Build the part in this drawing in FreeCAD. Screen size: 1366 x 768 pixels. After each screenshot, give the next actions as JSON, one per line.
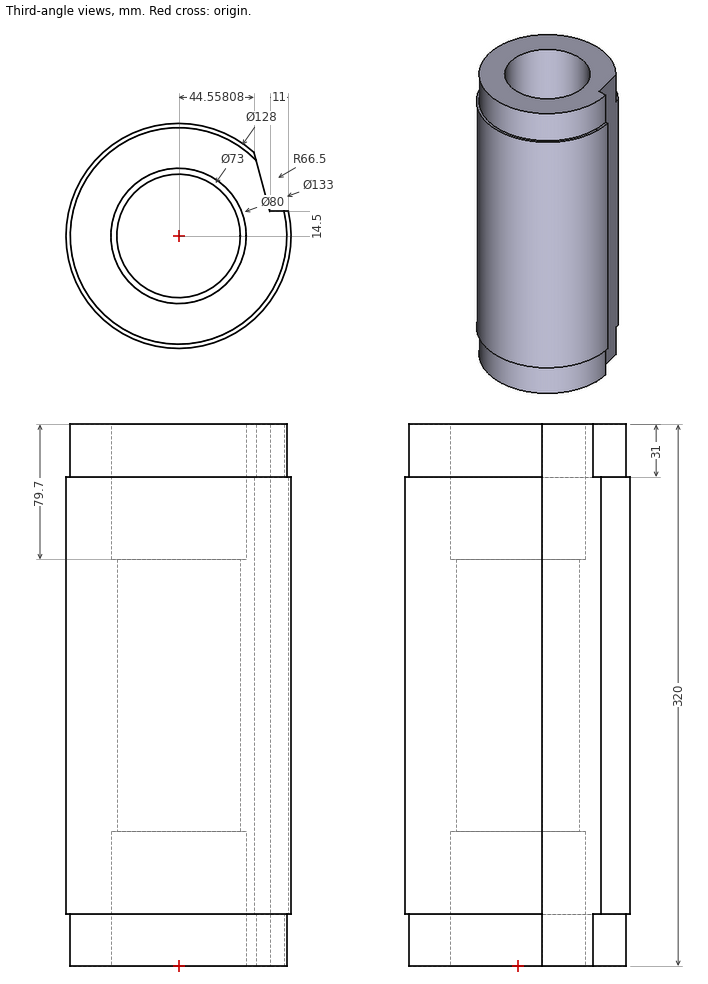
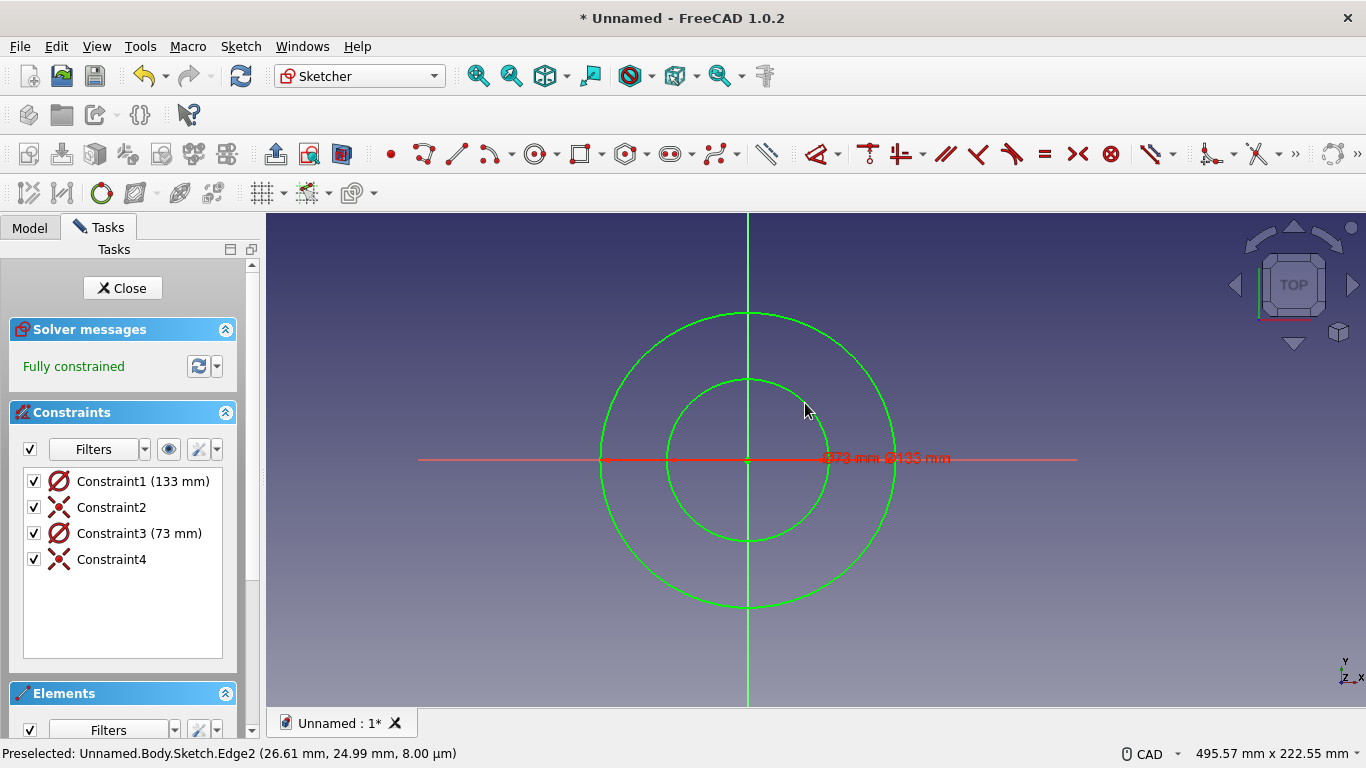
{"action": "left_click", "coordinate": [123, 288]}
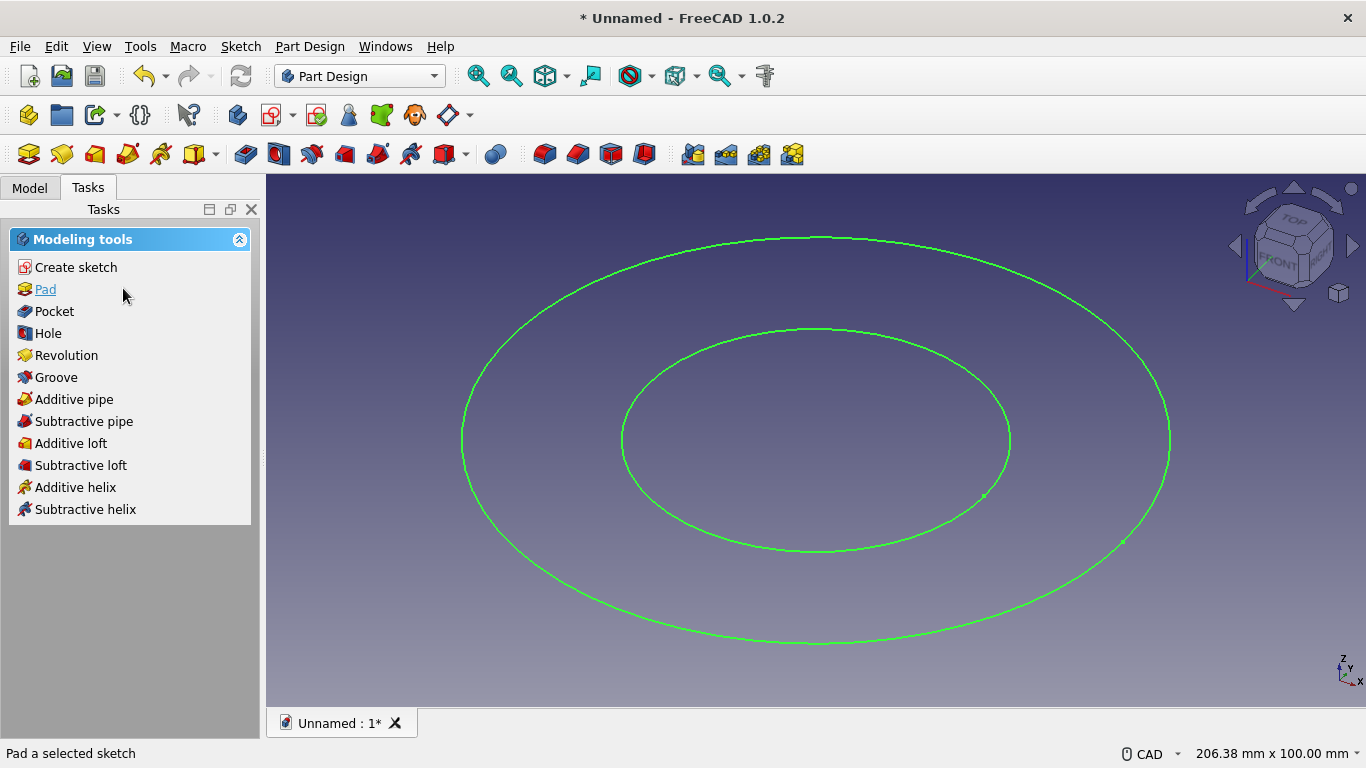
{"action": "left_click", "coordinate": [29, 154]}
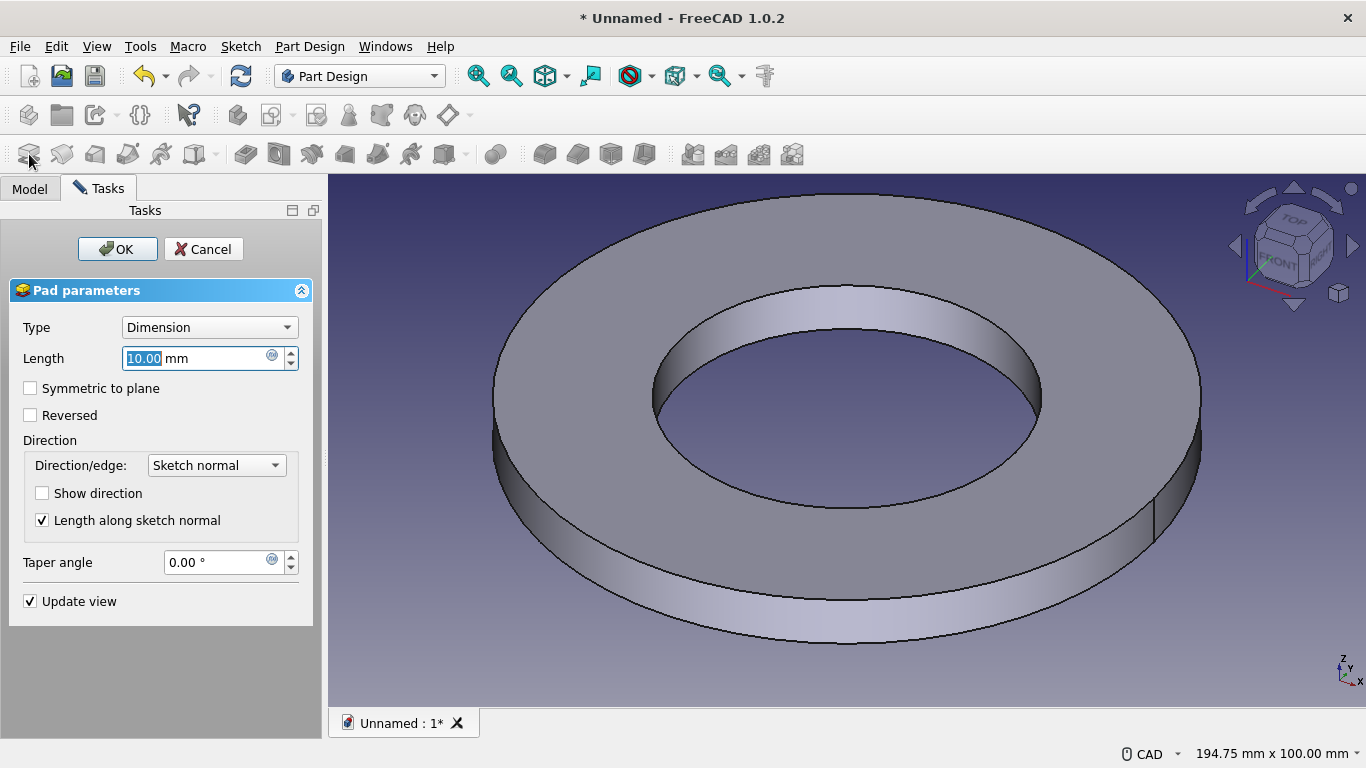
{"action": "type", "text": "320"}
{"action": "key", "text": "Tab"}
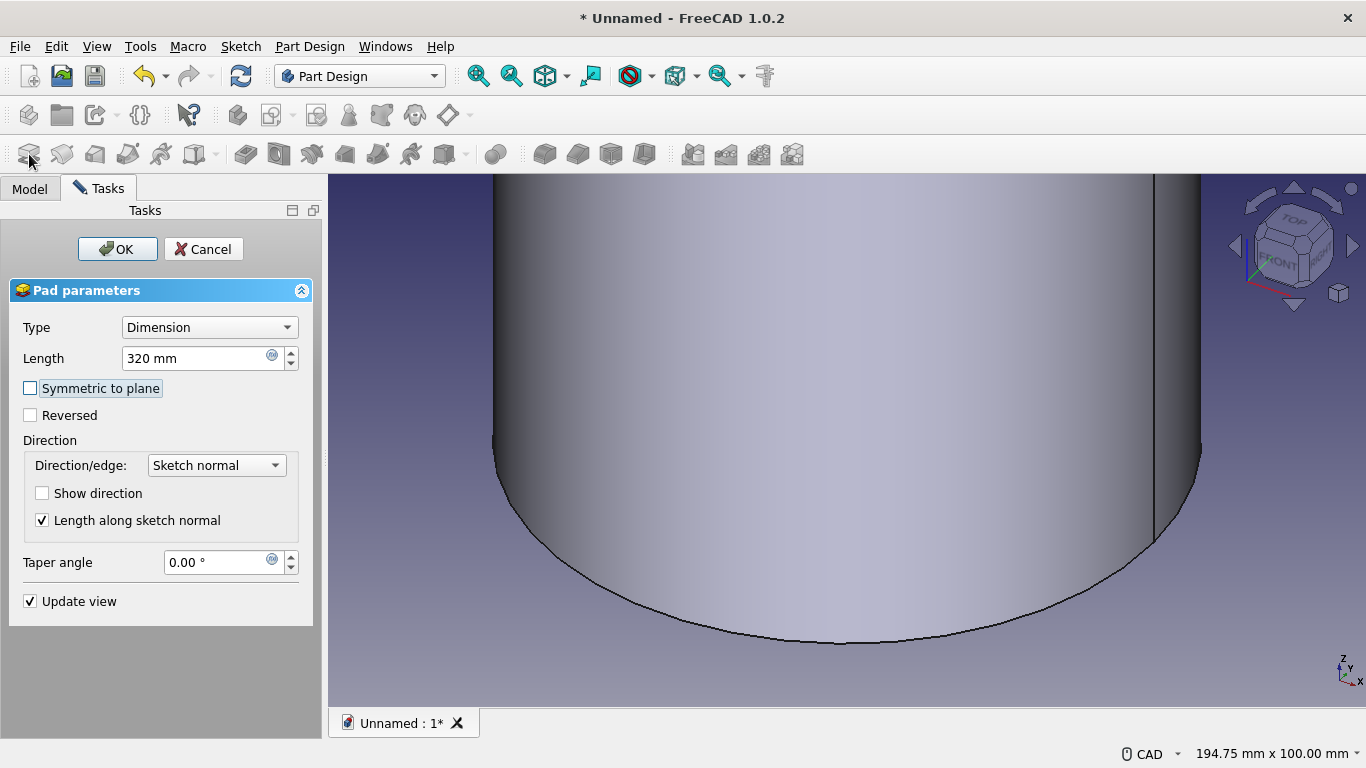
{"action": "left_click", "coordinate": [118, 249]}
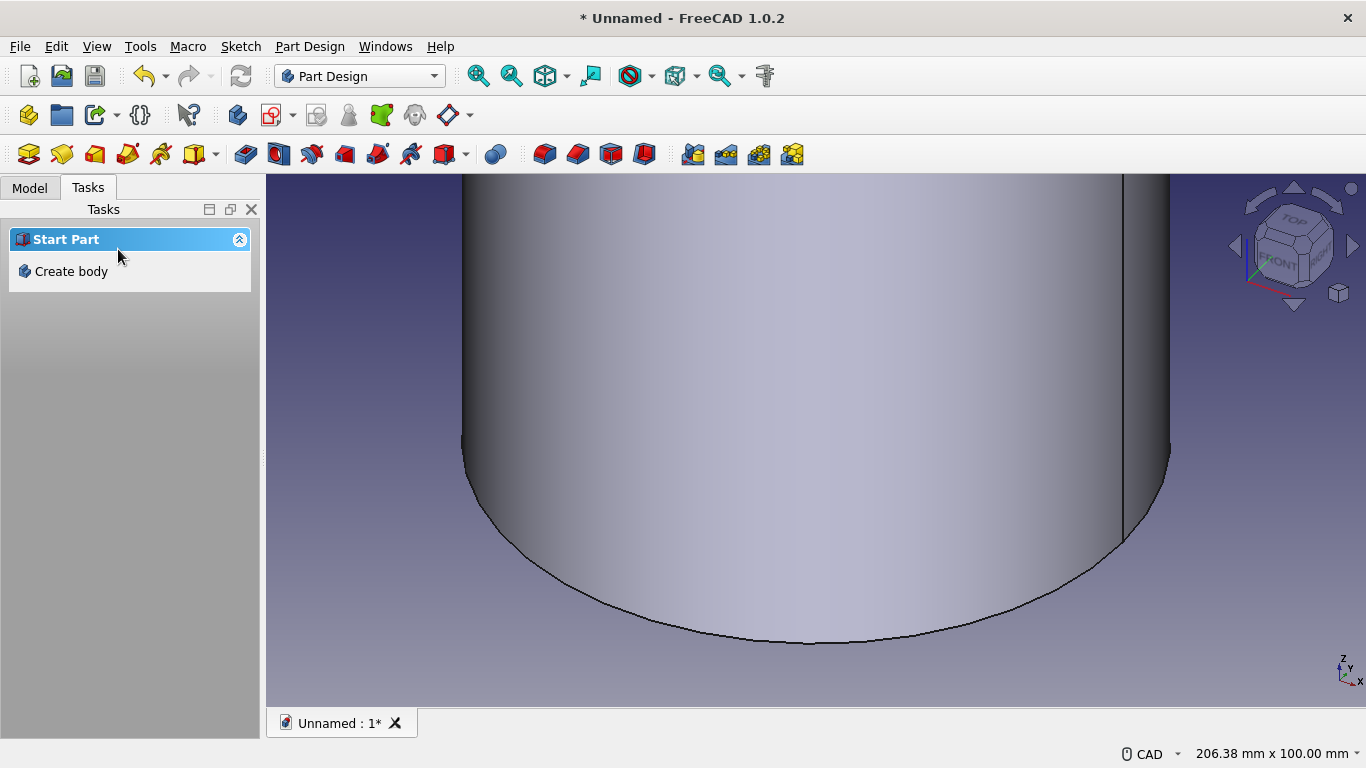
{"action": "left_click", "coordinate": [479, 76]}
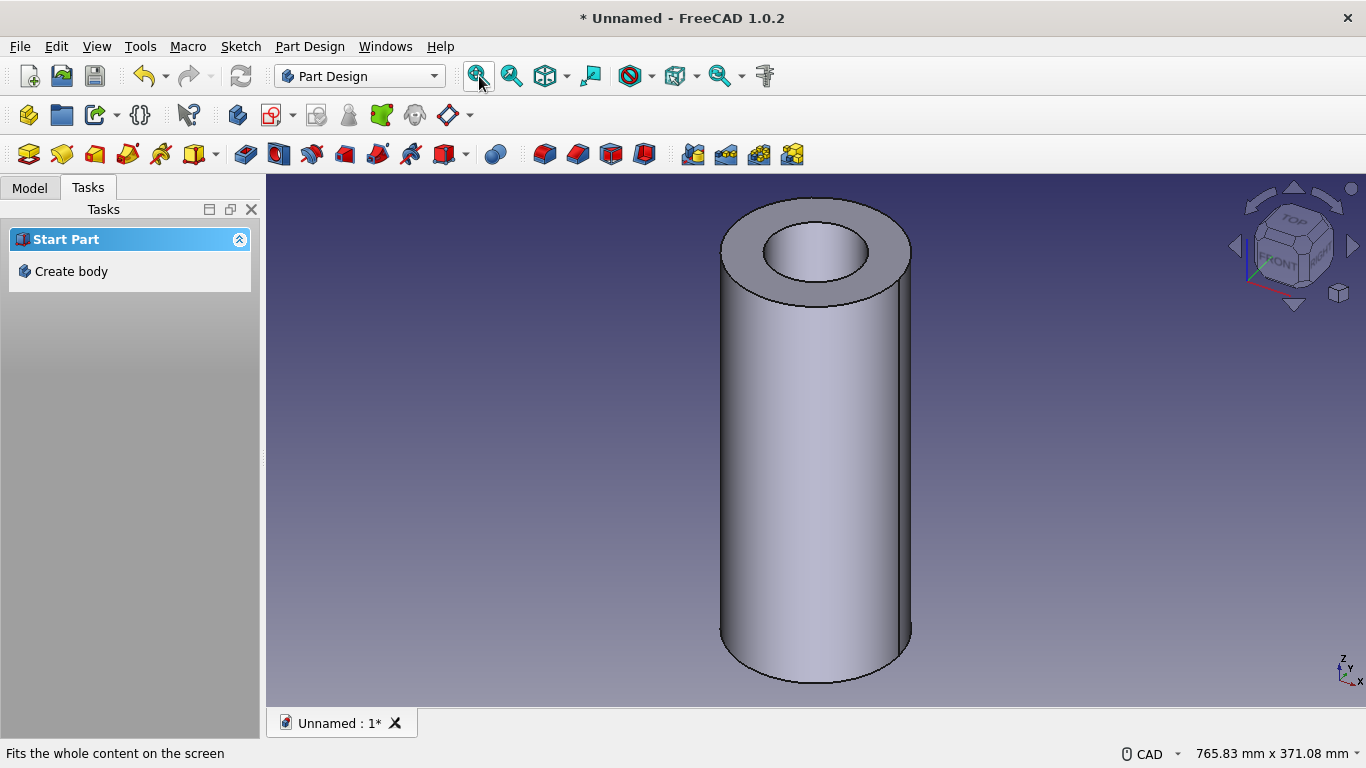
{"action": "left_click", "coordinate": [741, 263]}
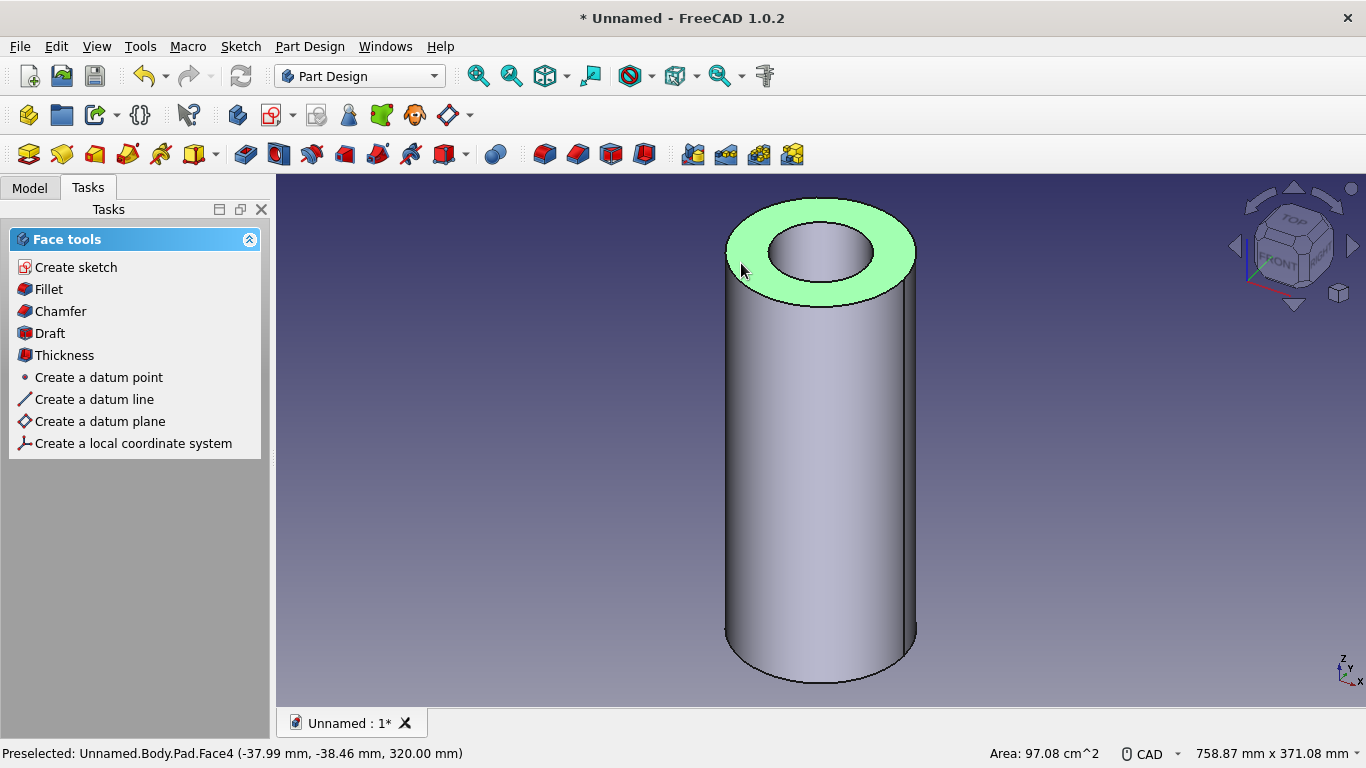
{"action": "left_click", "coordinate": [270, 116]}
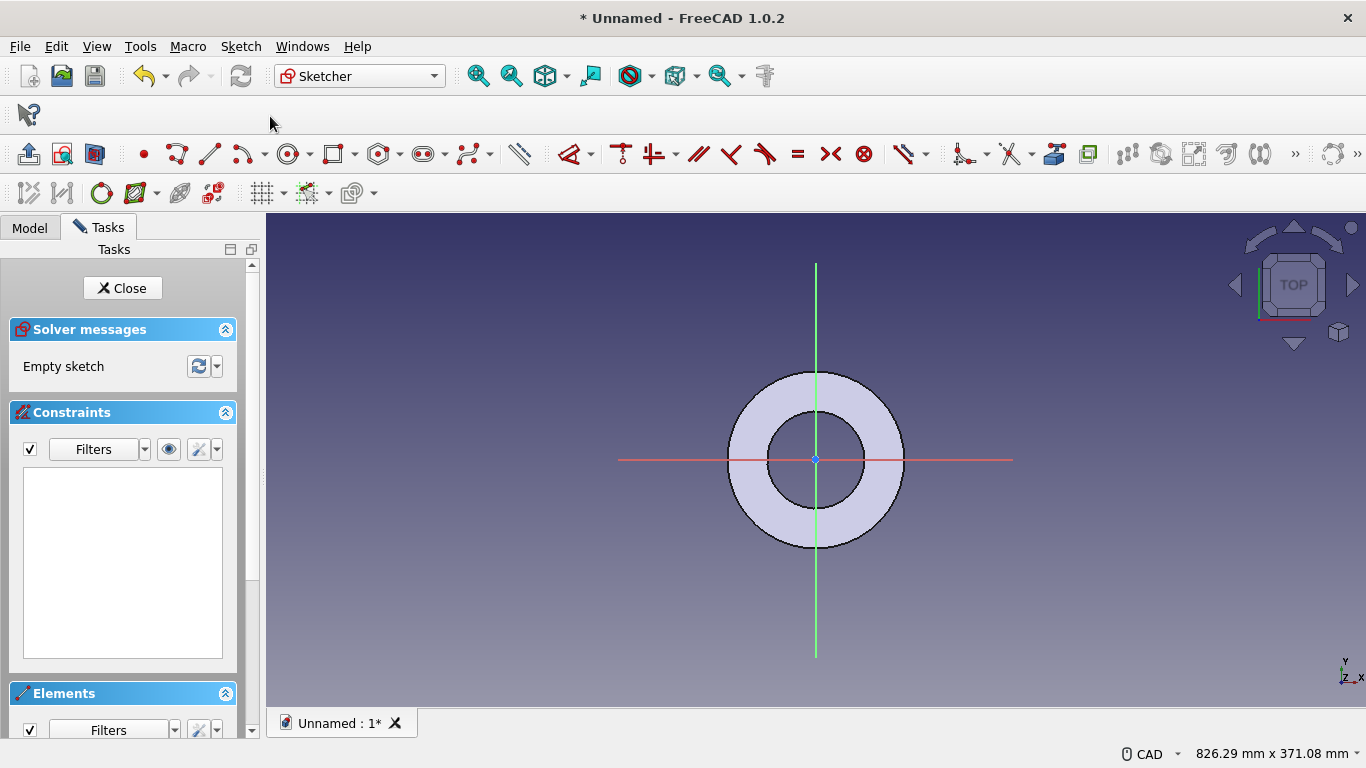
{"action": "scroll", "coordinate": [856, 460], "scroll_direction": "up", "scroll_amount": 5}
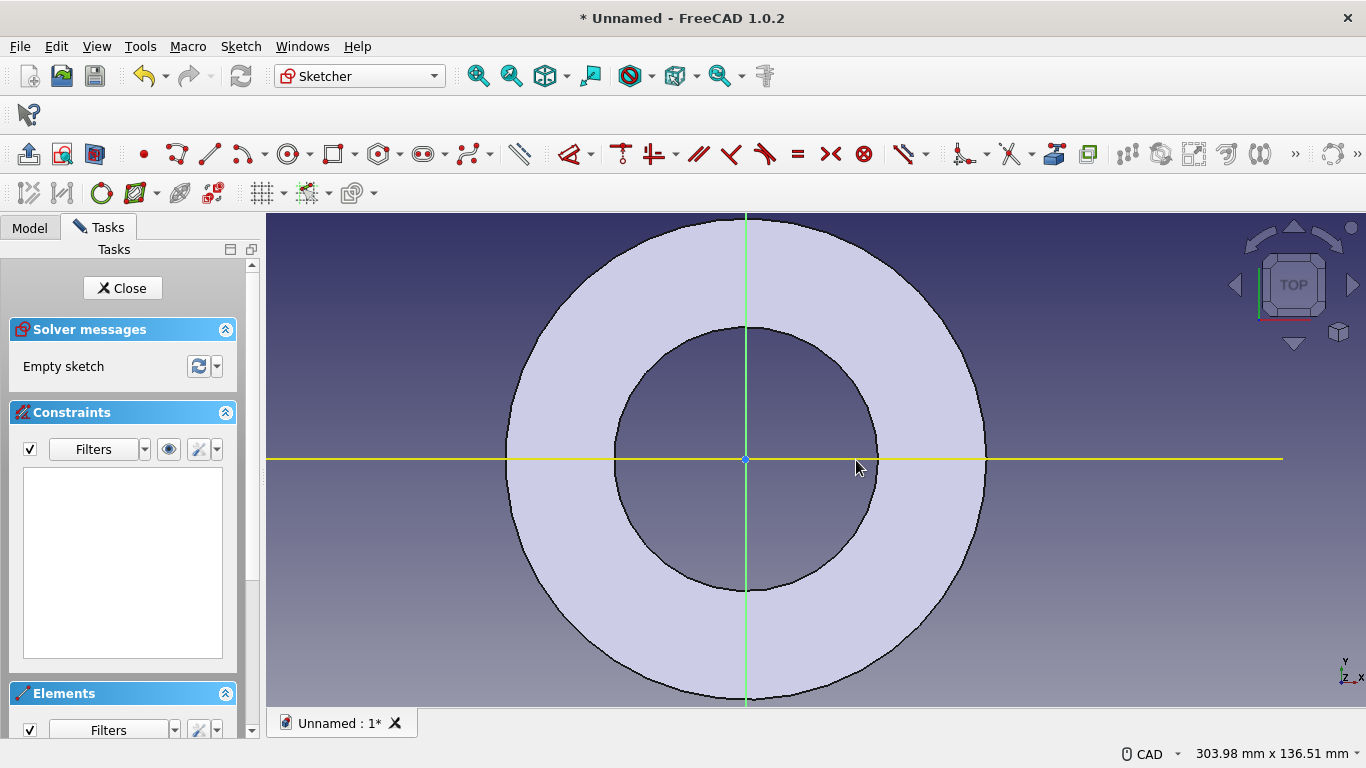
{"action": "left_click", "coordinate": [288, 154]}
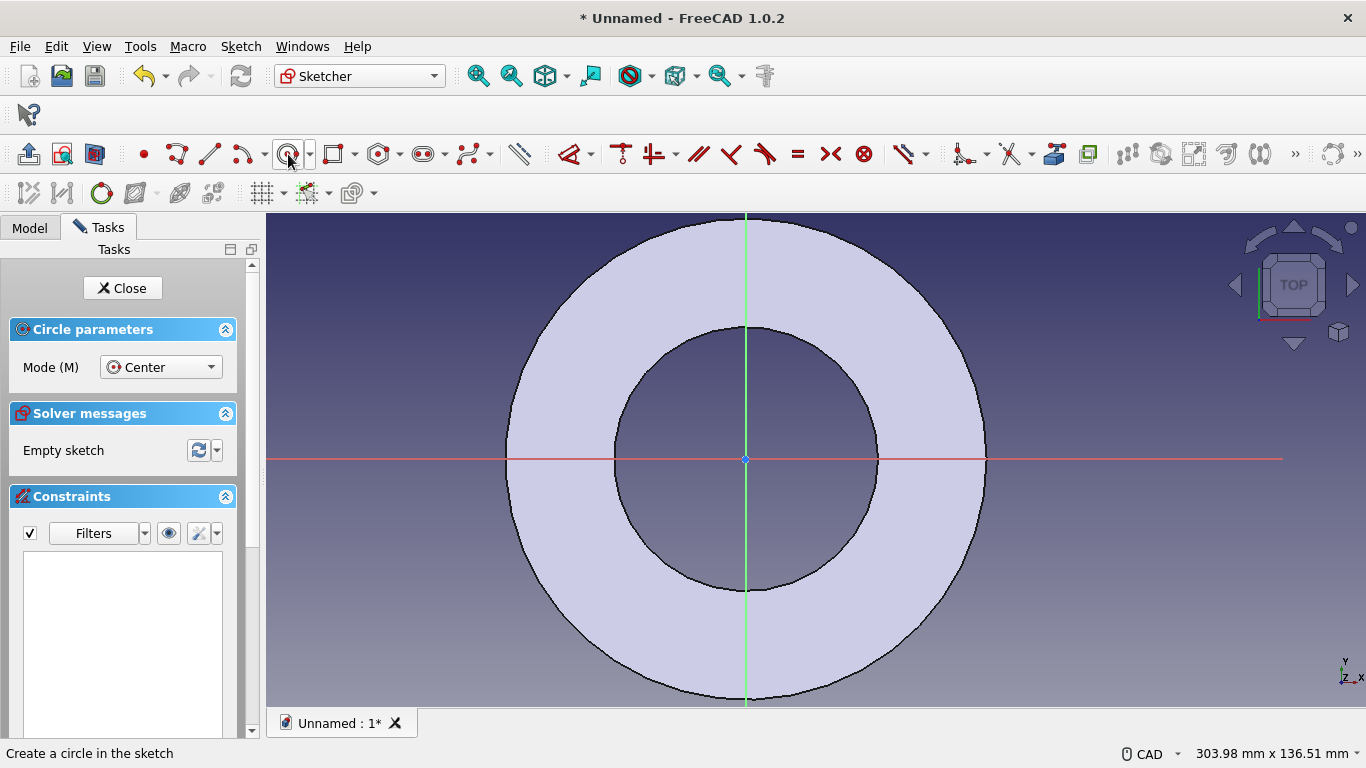
{"action": "left_click", "coordinate": [746, 459]}
{"action": "mouse_move", "coordinate": [848, 357]}